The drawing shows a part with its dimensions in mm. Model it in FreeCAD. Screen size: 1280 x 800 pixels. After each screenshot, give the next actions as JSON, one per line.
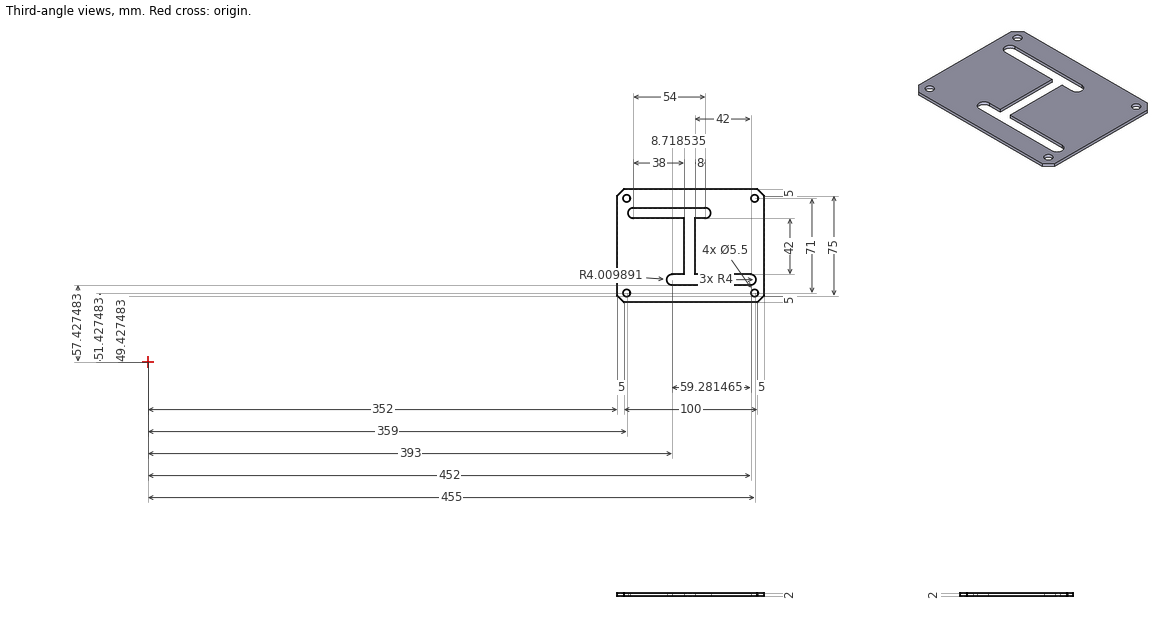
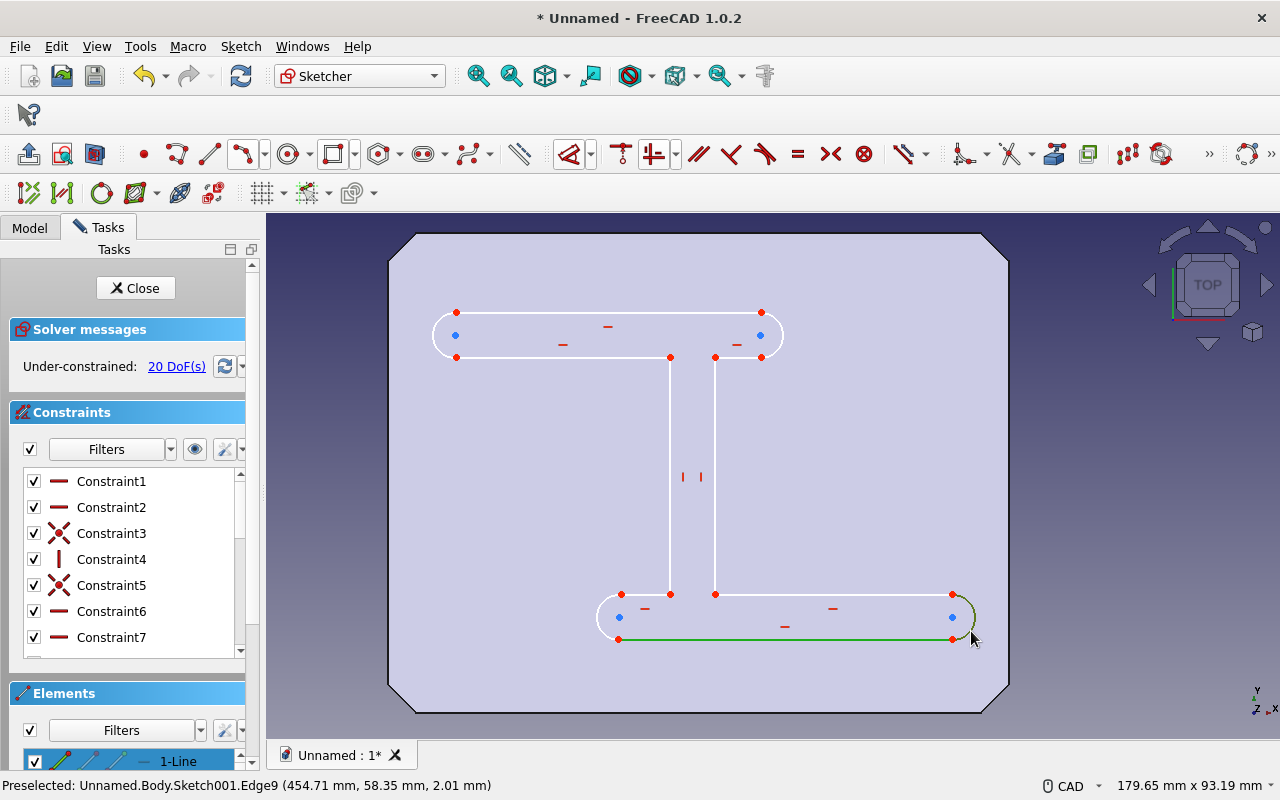
{"action": "left_click", "coordinate": [765, 154]}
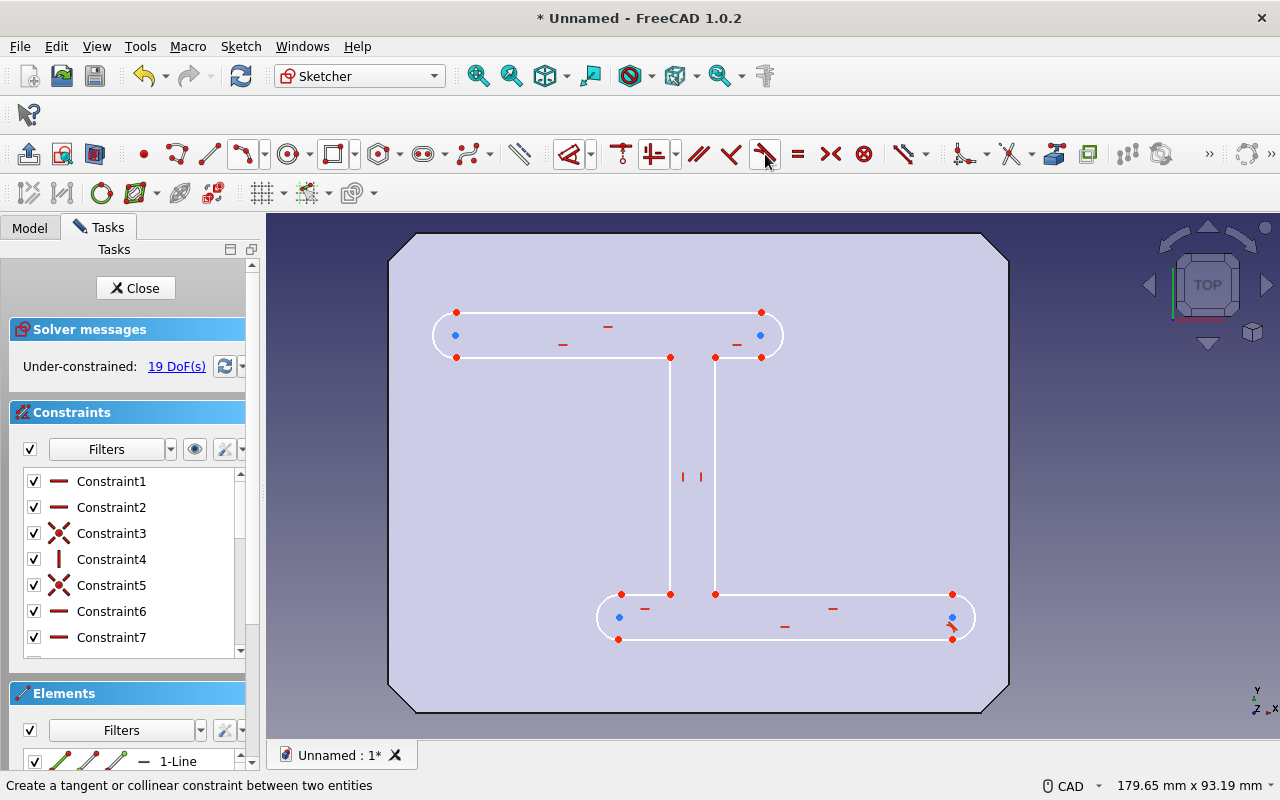
{"action": "left_click", "coordinate": [881, 595]}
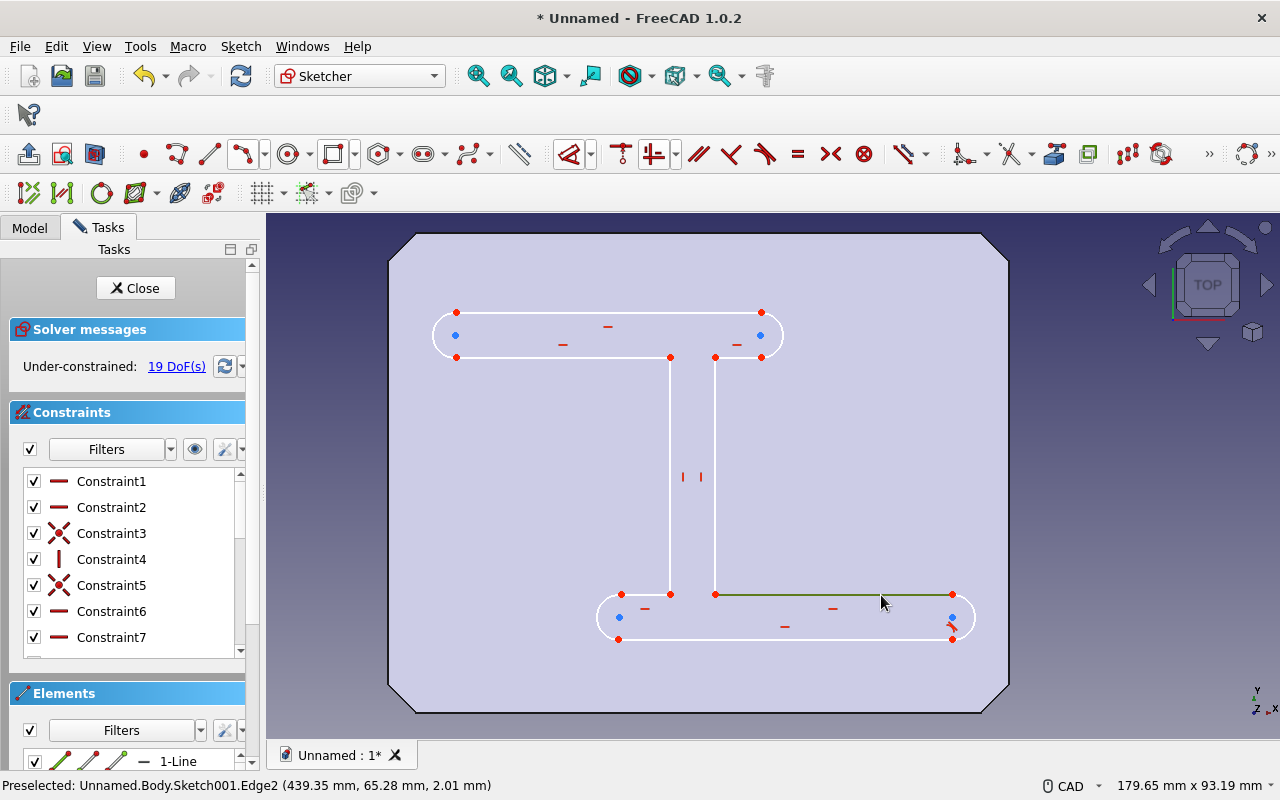
{"action": "left_click", "coordinate": [971, 631]}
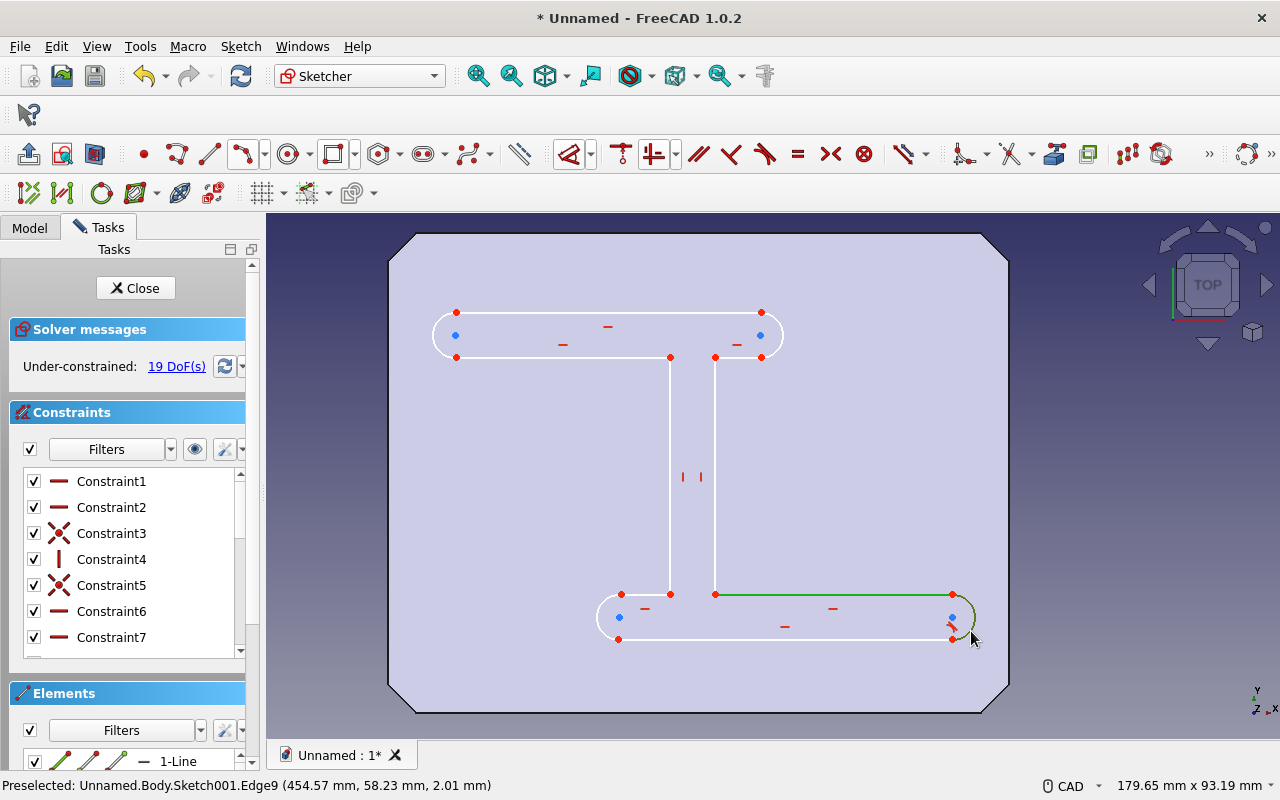
{"action": "left_click", "coordinate": [765, 154]}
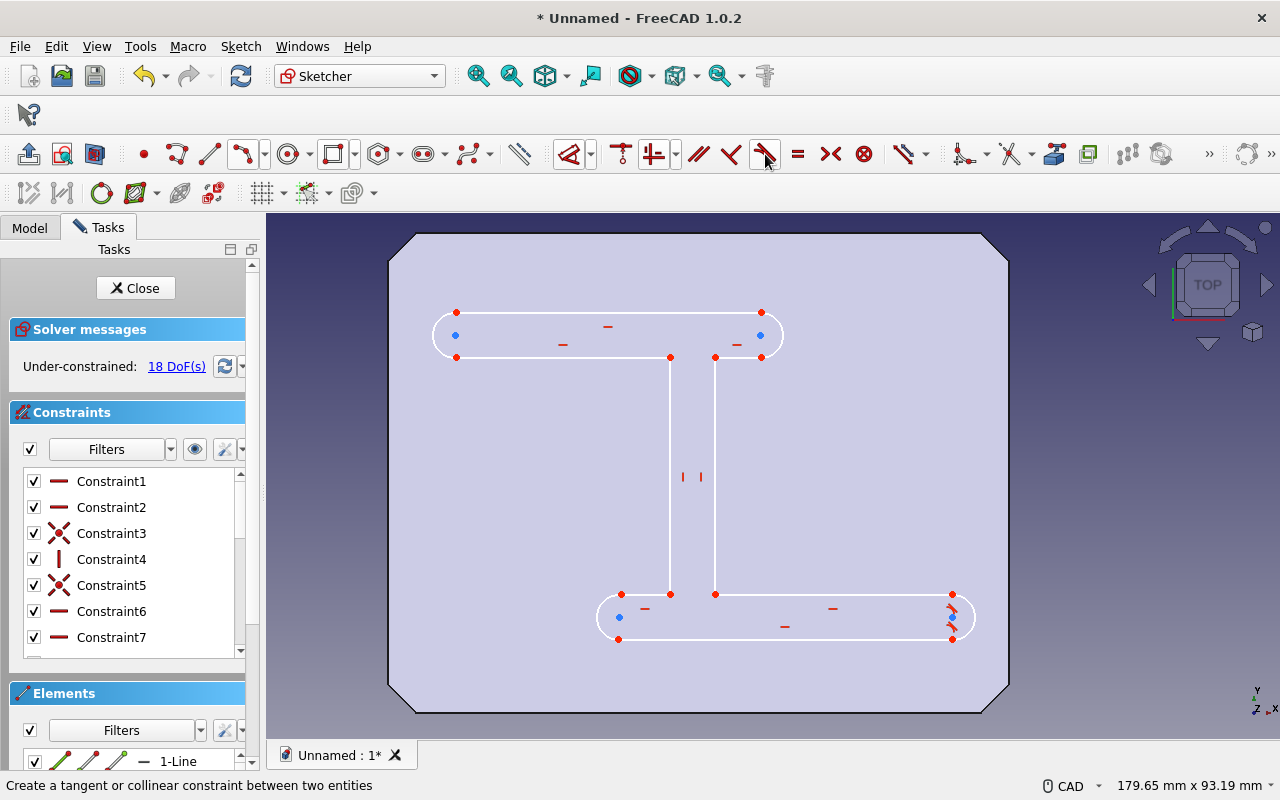
{"action": "left_click", "coordinate": [729, 358]}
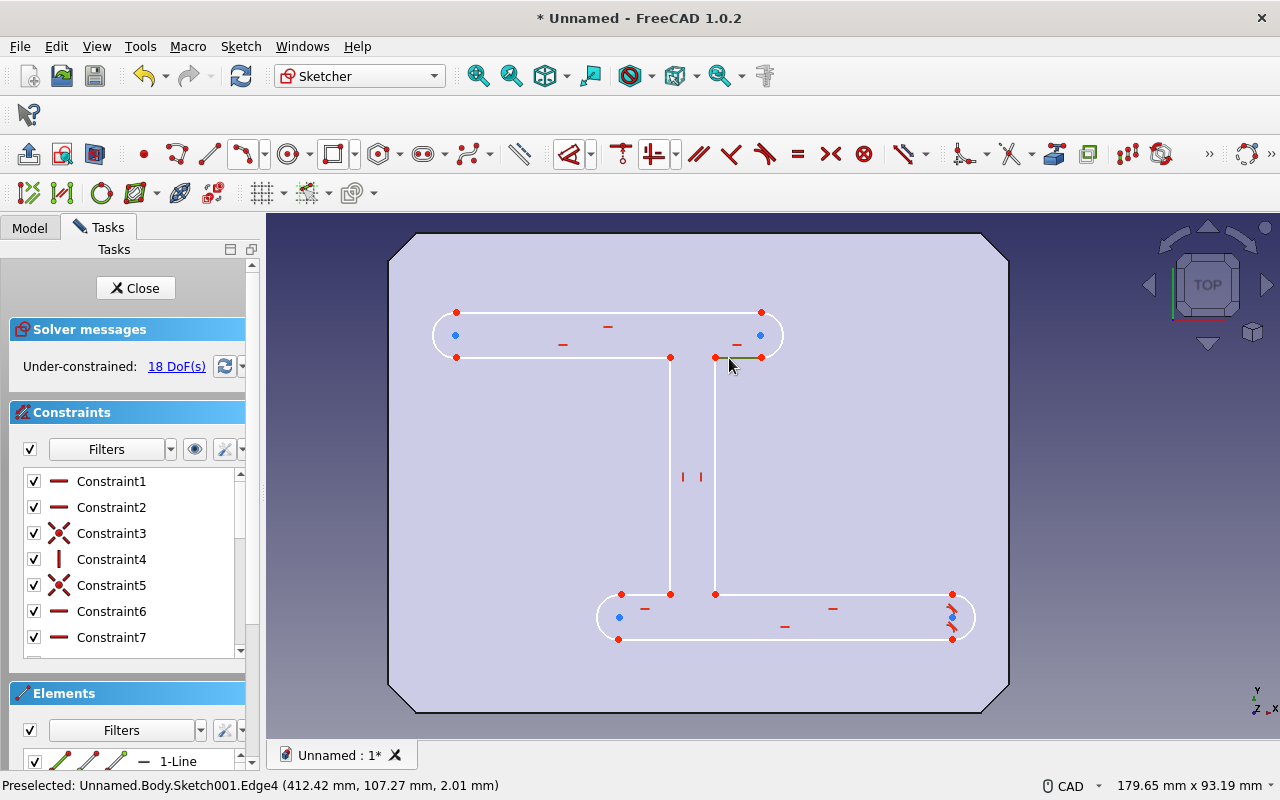
{"action": "left_click", "coordinate": [779, 349]}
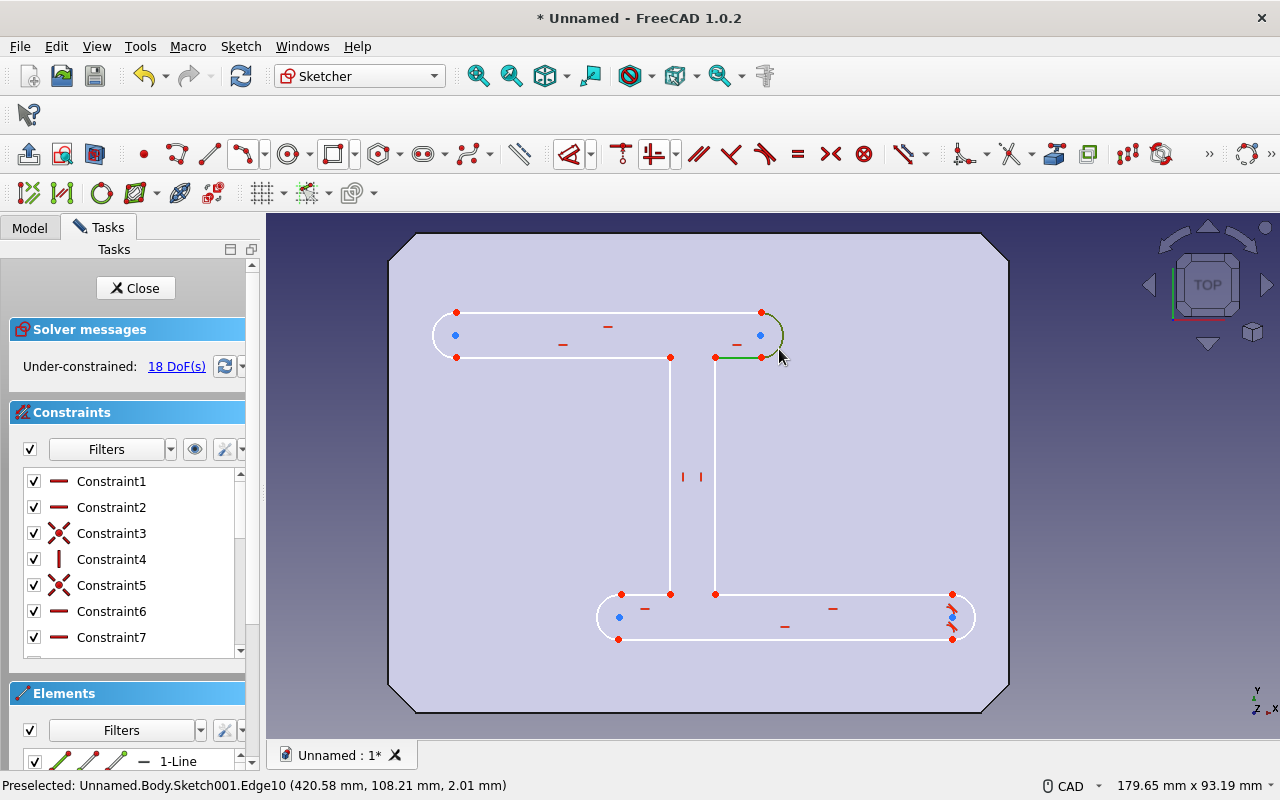
{"action": "left_click", "coordinate": [765, 154]}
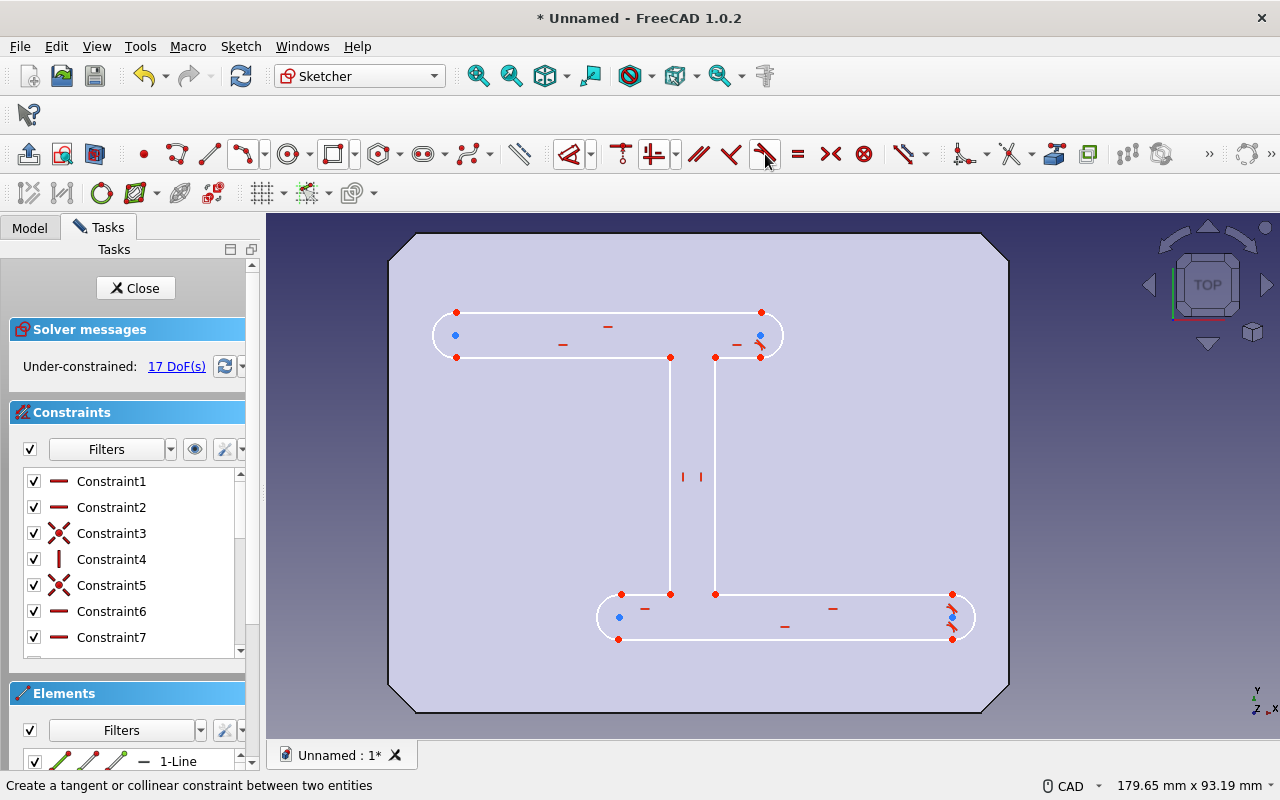
{"action": "left_click", "coordinate": [669, 313]}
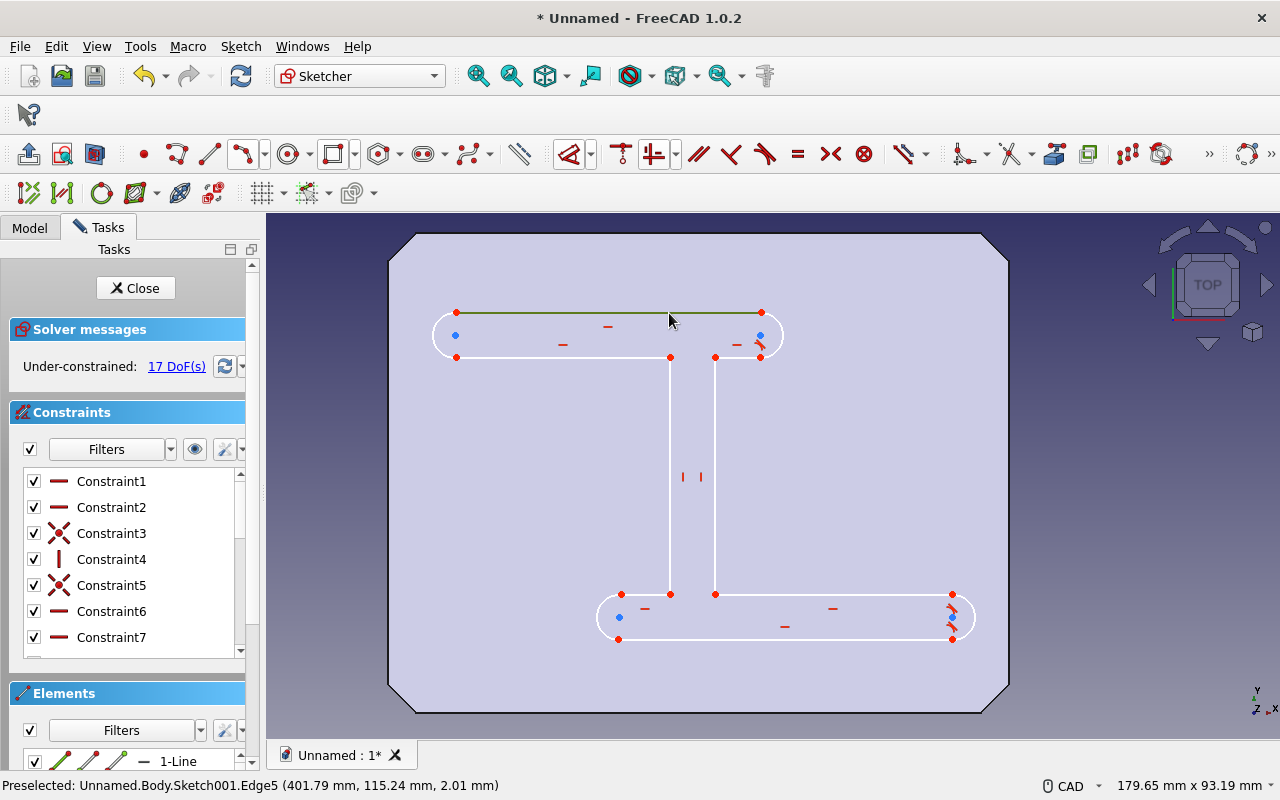
{"action": "left_click", "coordinate": [779, 349]}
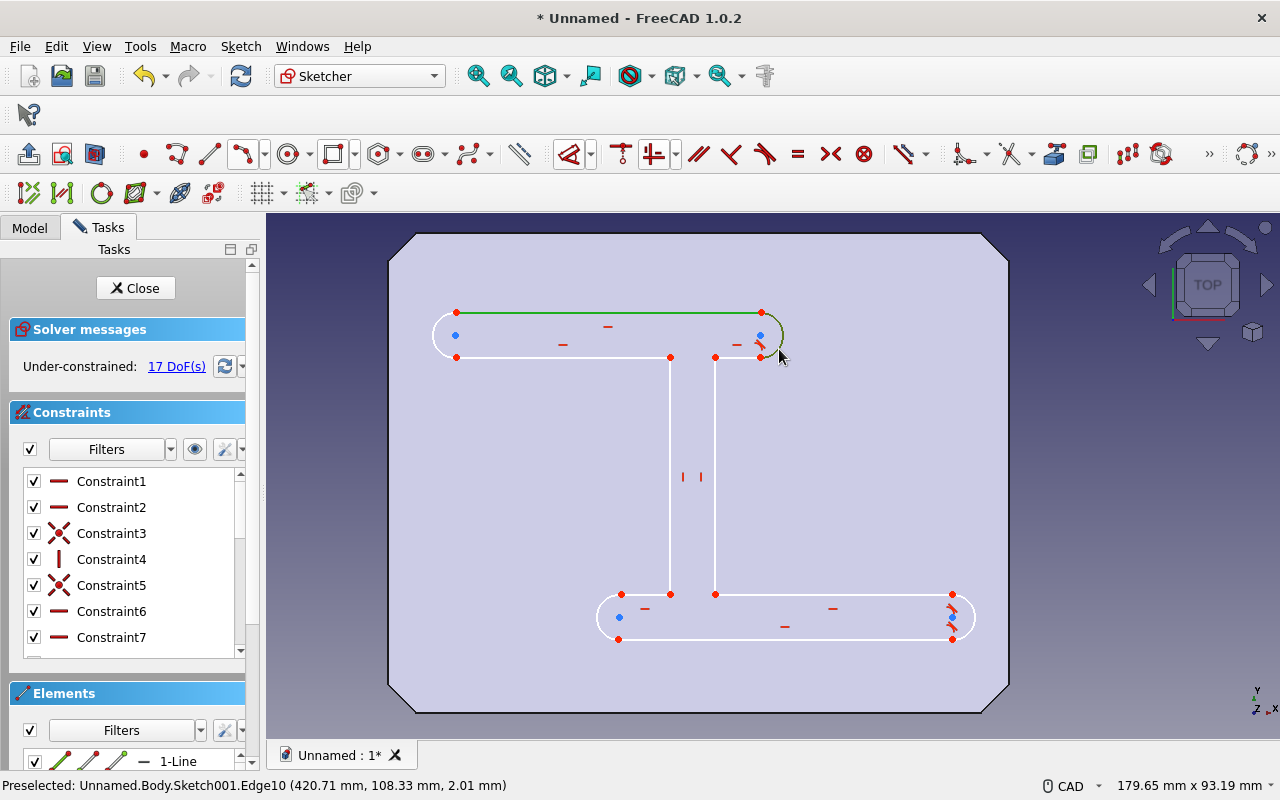
{"action": "left_click", "coordinate": [765, 154]}